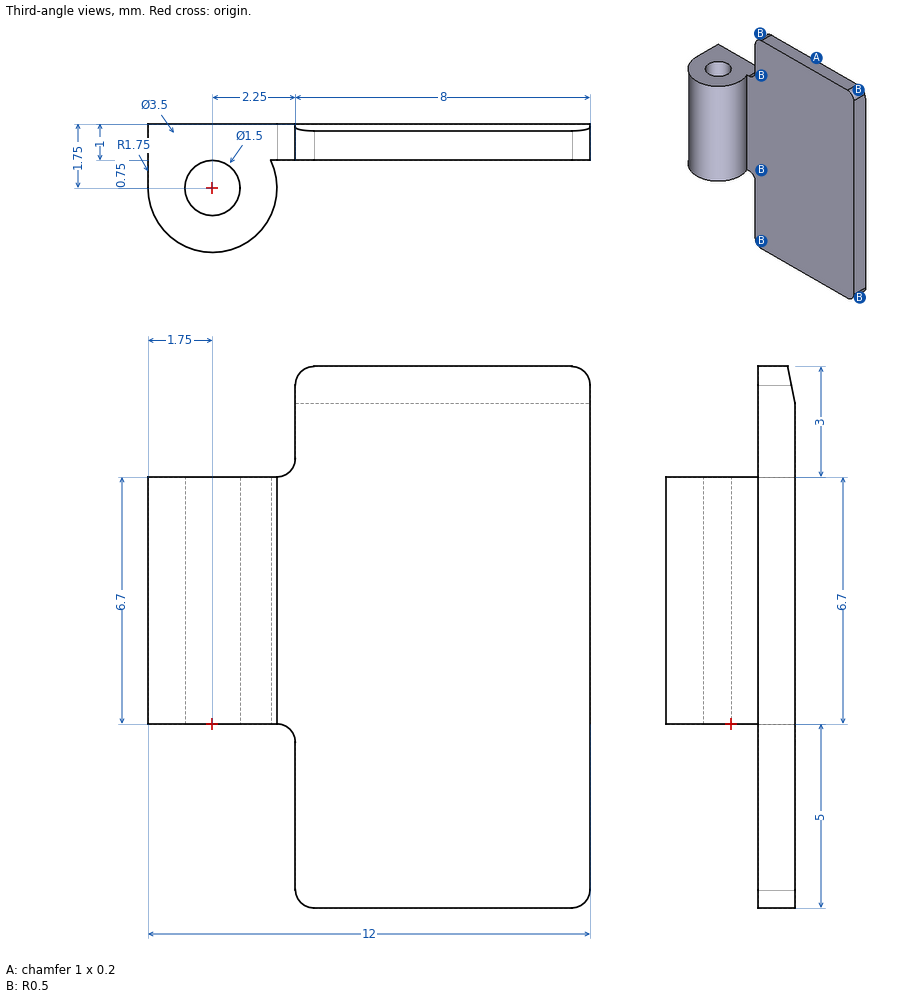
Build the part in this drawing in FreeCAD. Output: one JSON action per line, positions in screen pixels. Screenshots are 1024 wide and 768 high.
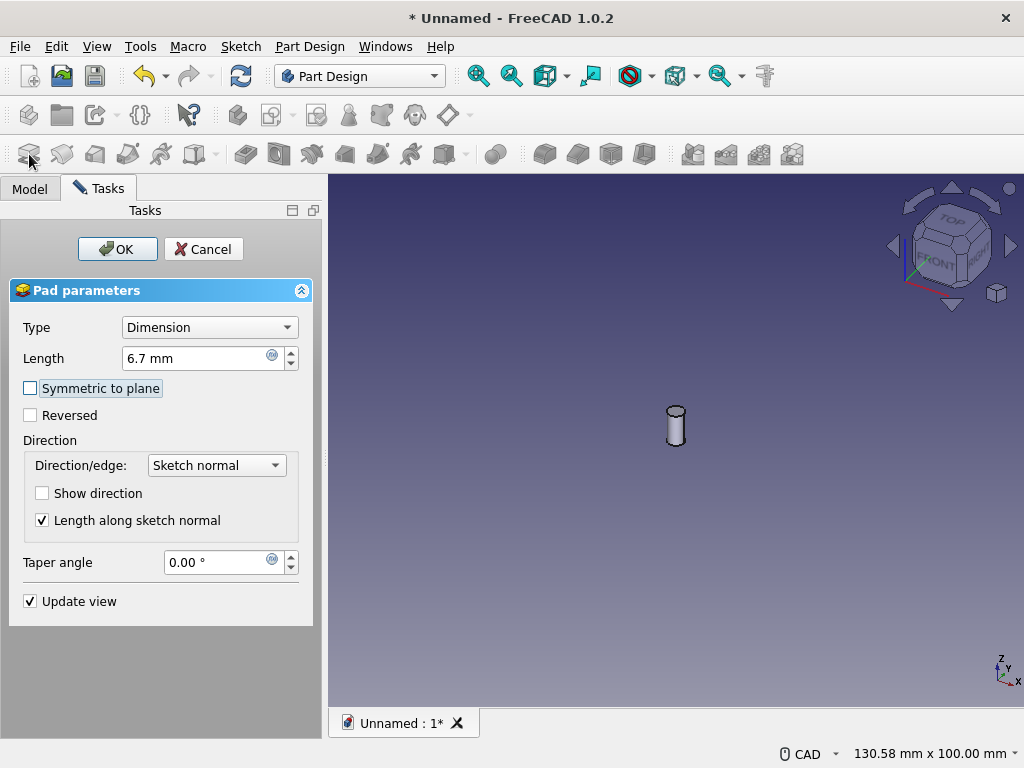
{"action": "left_click", "coordinate": [118, 249]}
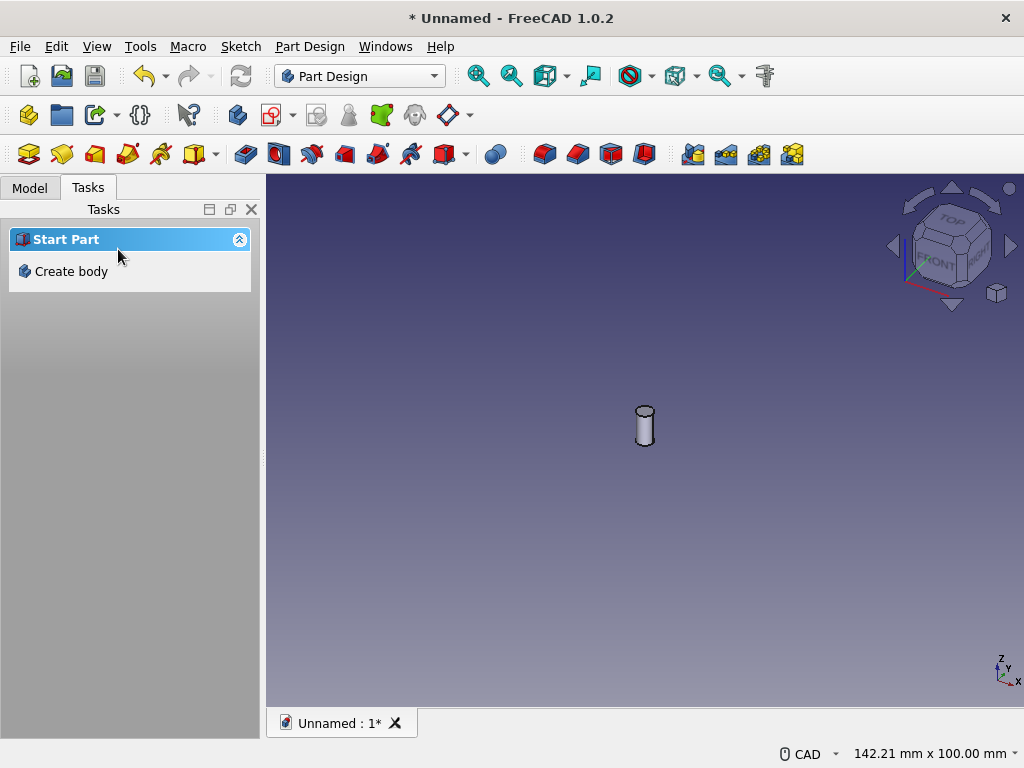
{"action": "left_click", "coordinate": [479, 76]}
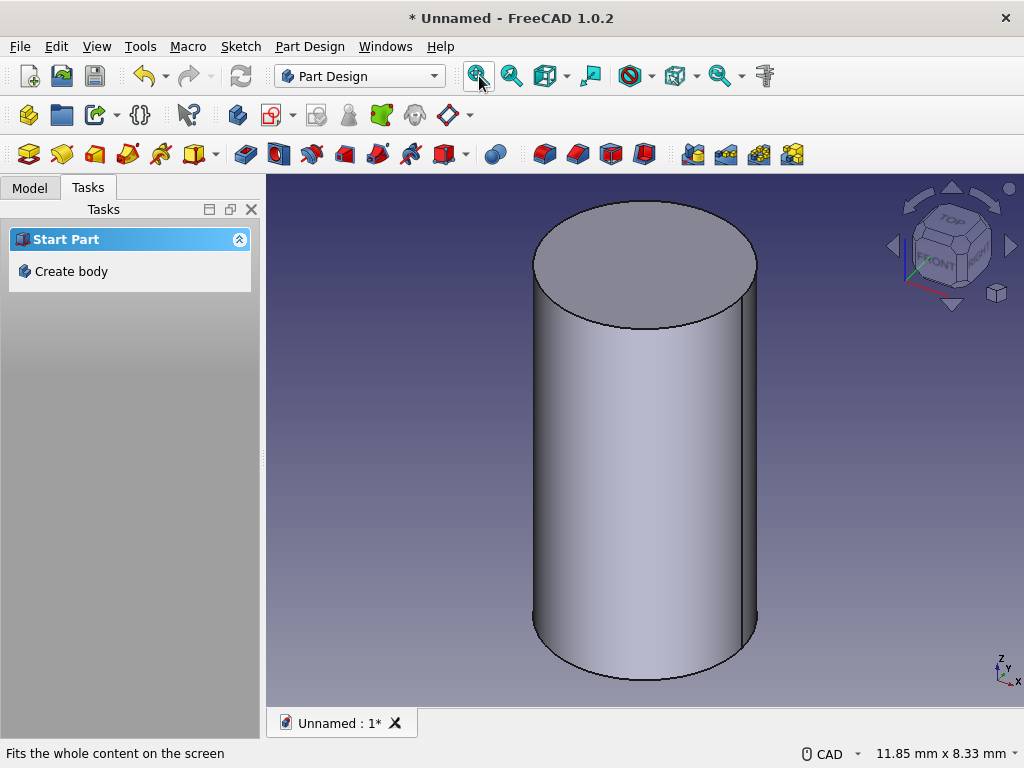
{"action": "left_click", "coordinate": [645, 264]}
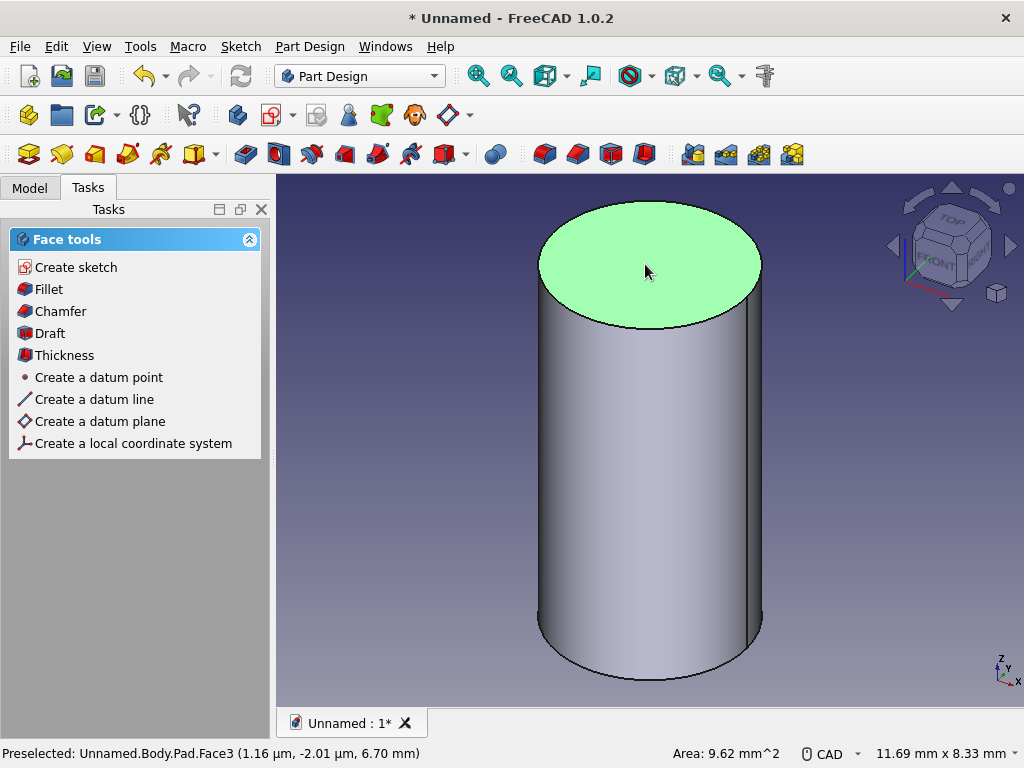
{"action": "left_click", "coordinate": [270, 116]}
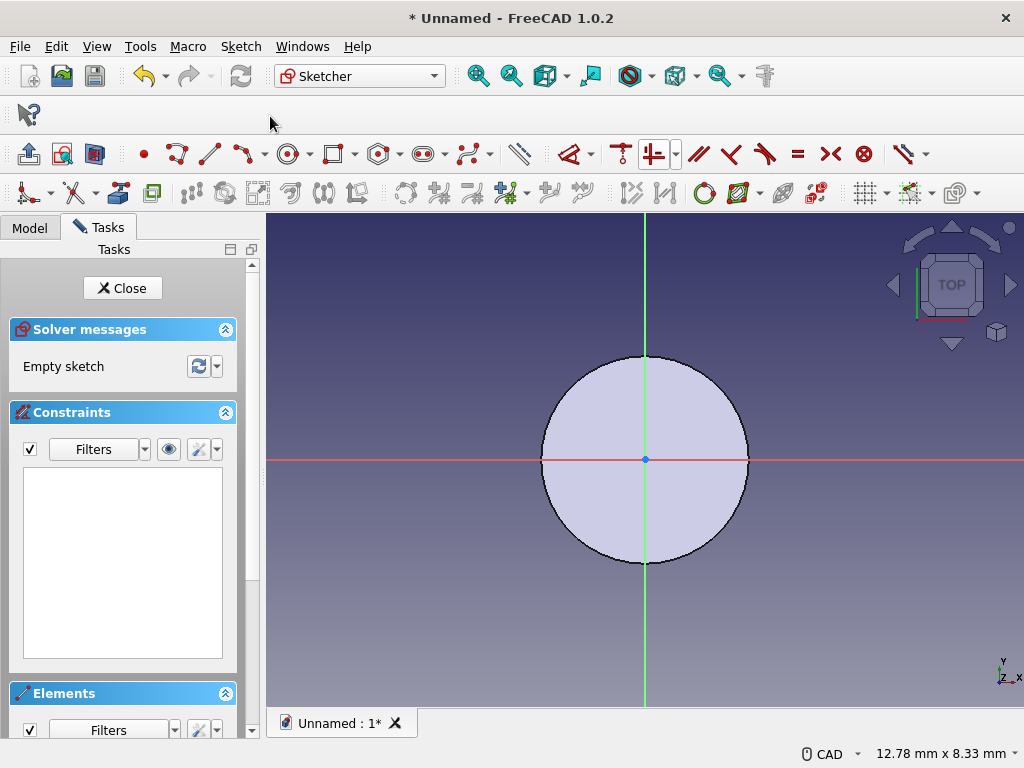
{"action": "scroll", "coordinate": [675, 460], "scroll_direction": "up", "scroll_amount": 6}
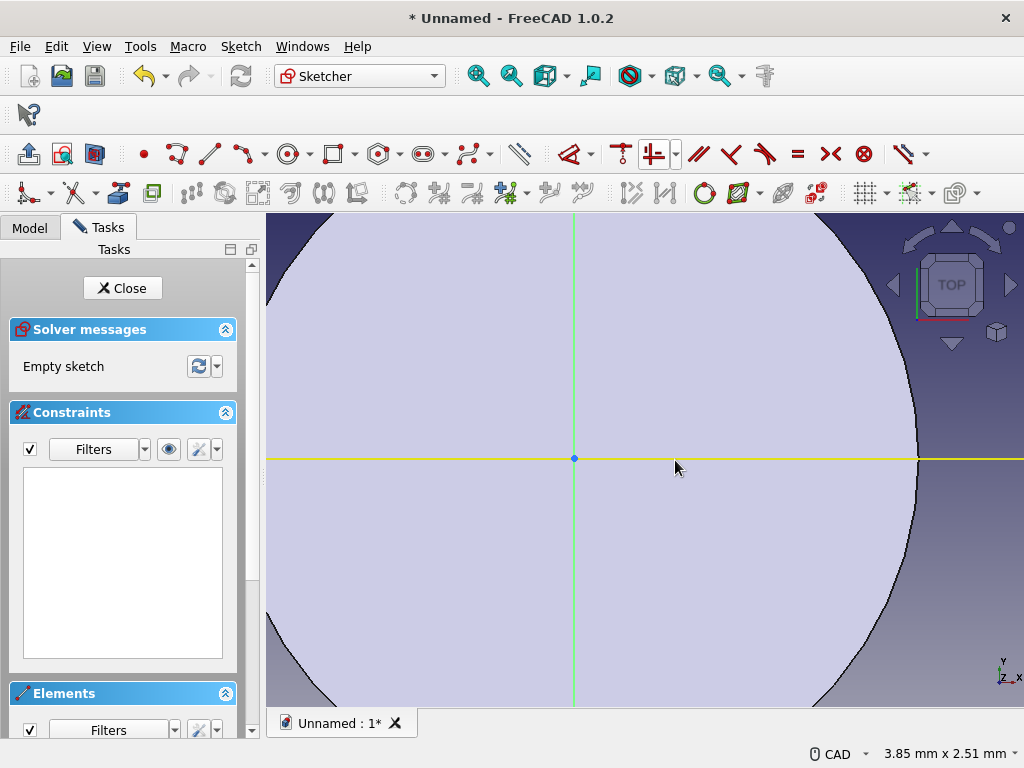
{"action": "left_click", "coordinate": [288, 154]}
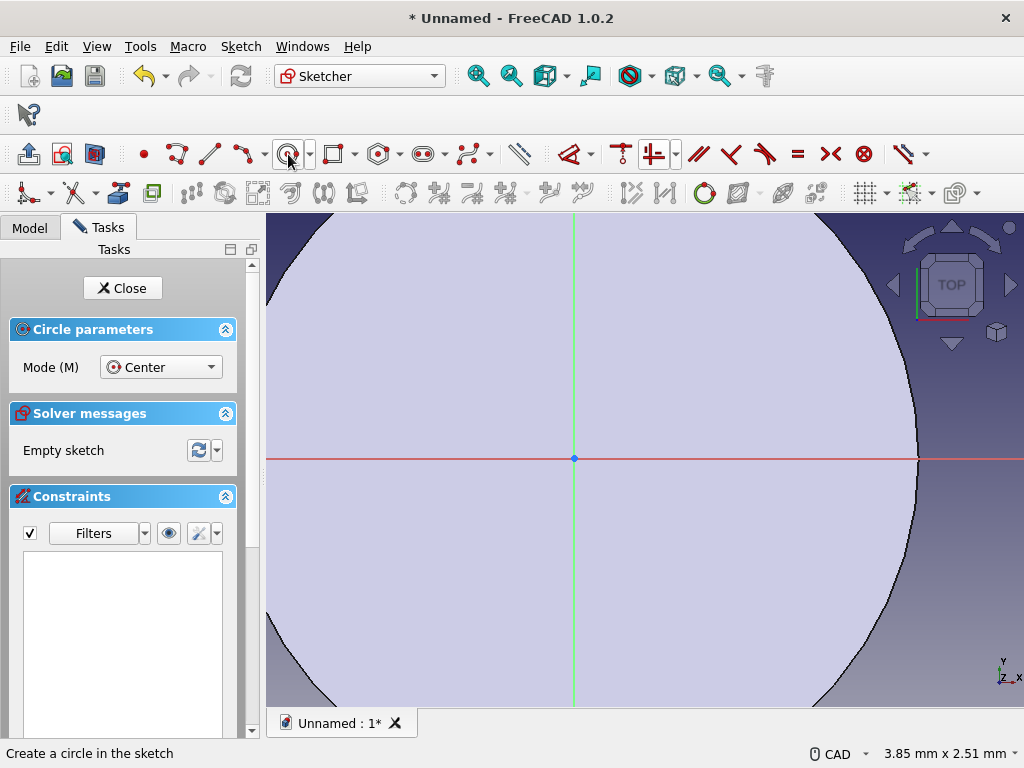
{"action": "left_click", "coordinate": [574, 459]}
{"action": "left_click", "coordinate": [679, 354]}
{"action": "key", "text": "Escape"}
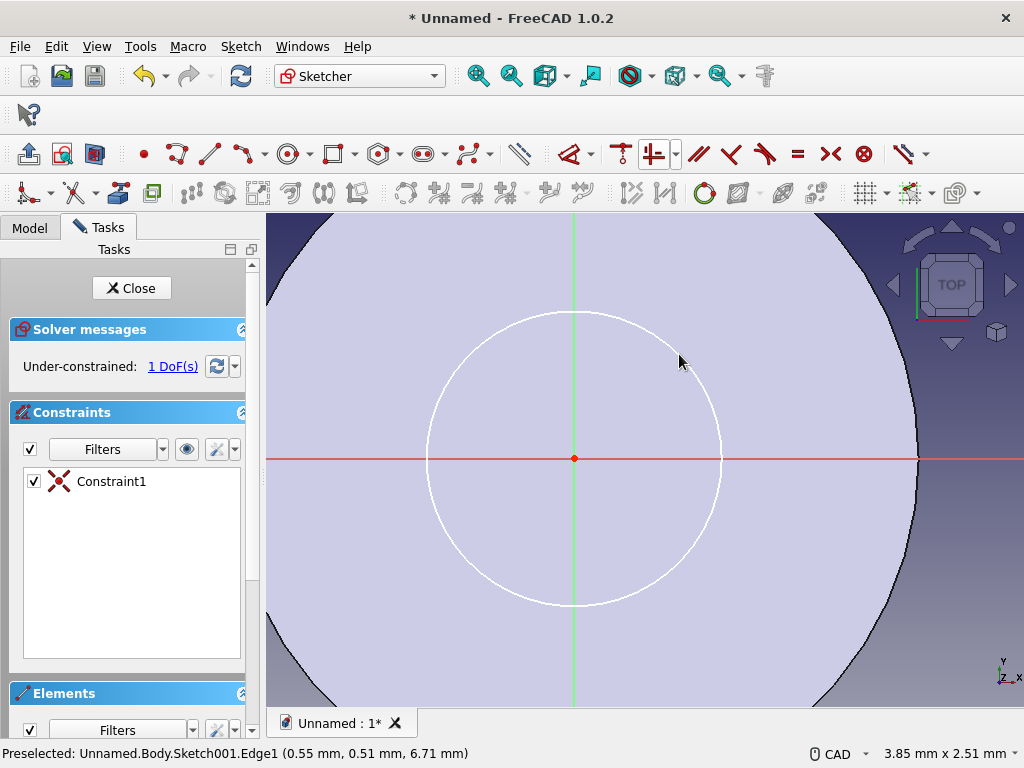
{"action": "left_click", "coordinate": [678, 354]}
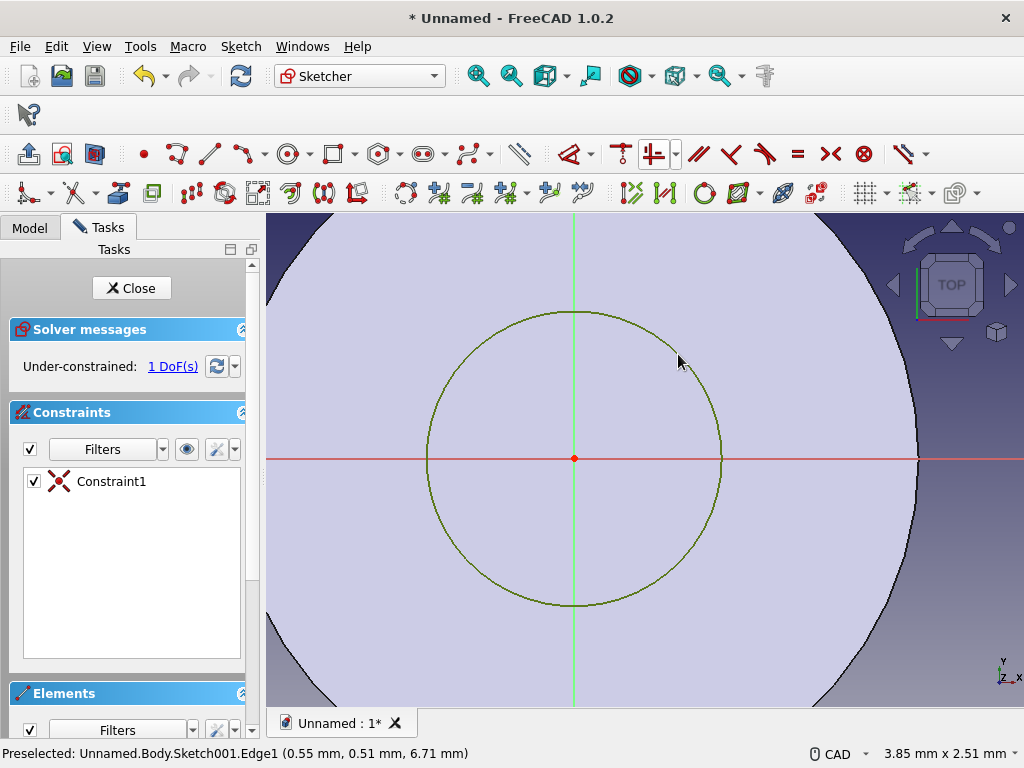
{"action": "left_click", "coordinate": [590, 154]}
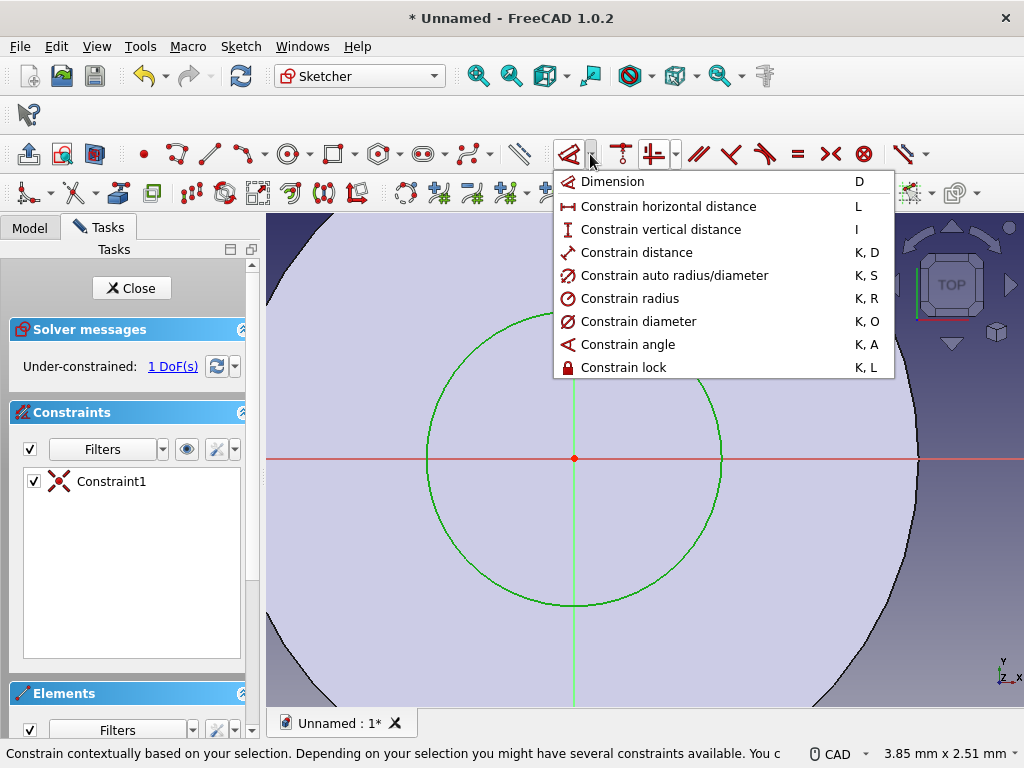
{"action": "left_click", "coordinate": [724, 322]}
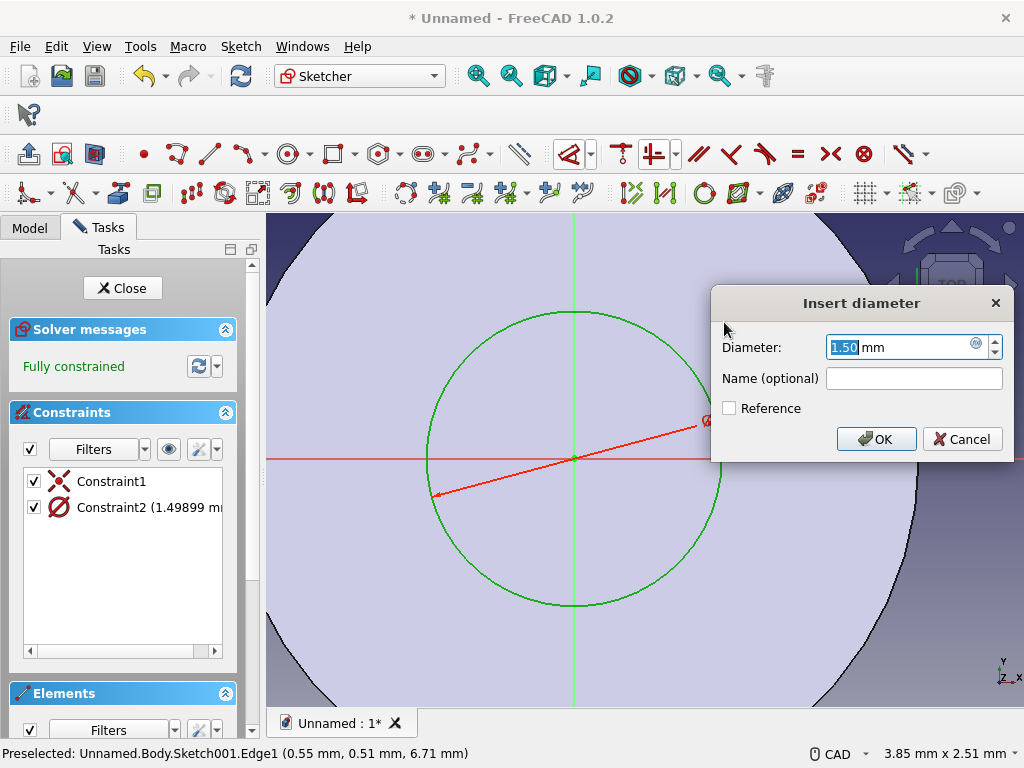
{"action": "type", "text": "1.5"}
{"action": "key", "text": "Return"}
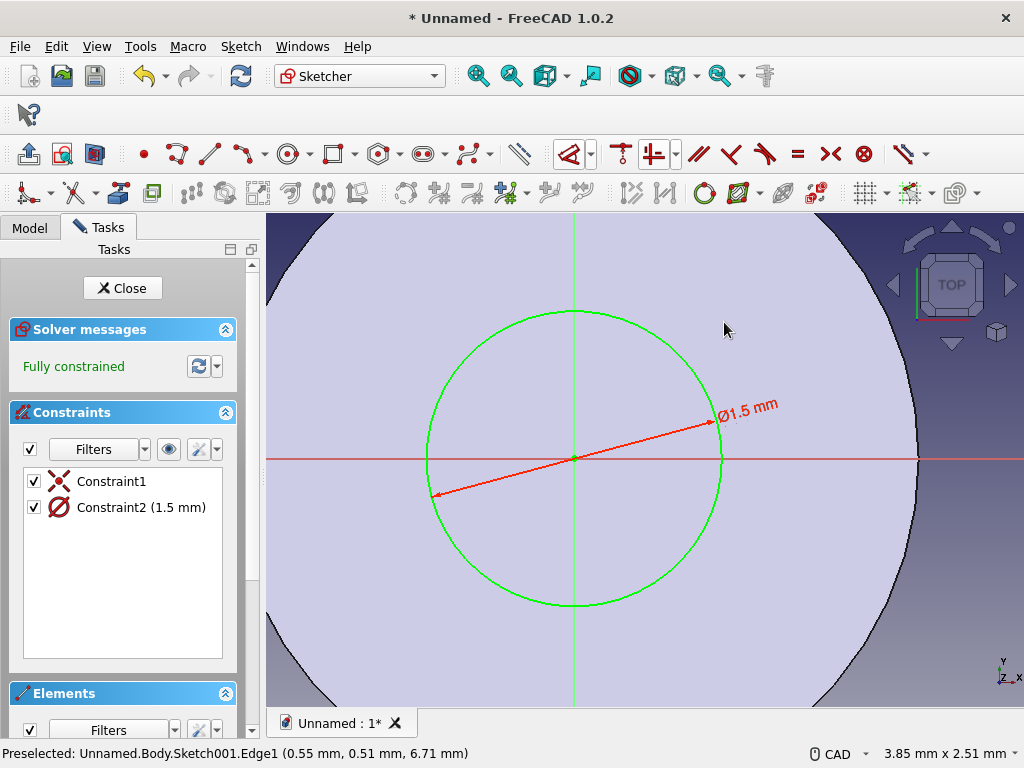
{"action": "left_click", "coordinate": [123, 288]}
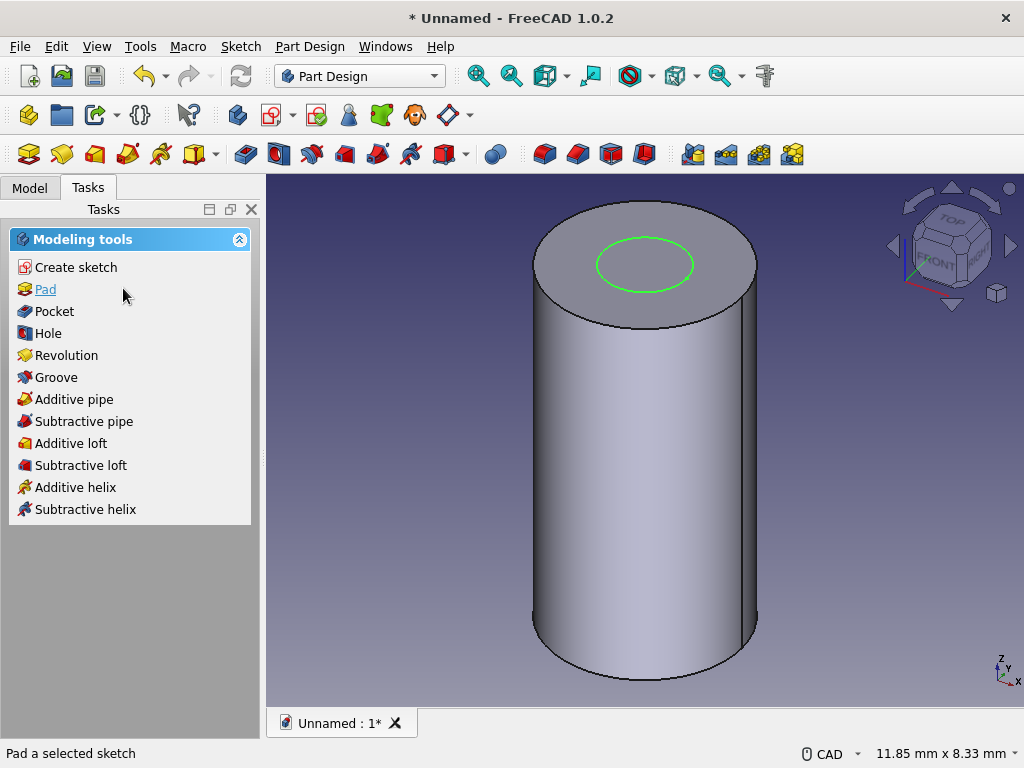
{"action": "left_click", "coordinate": [246, 154]}